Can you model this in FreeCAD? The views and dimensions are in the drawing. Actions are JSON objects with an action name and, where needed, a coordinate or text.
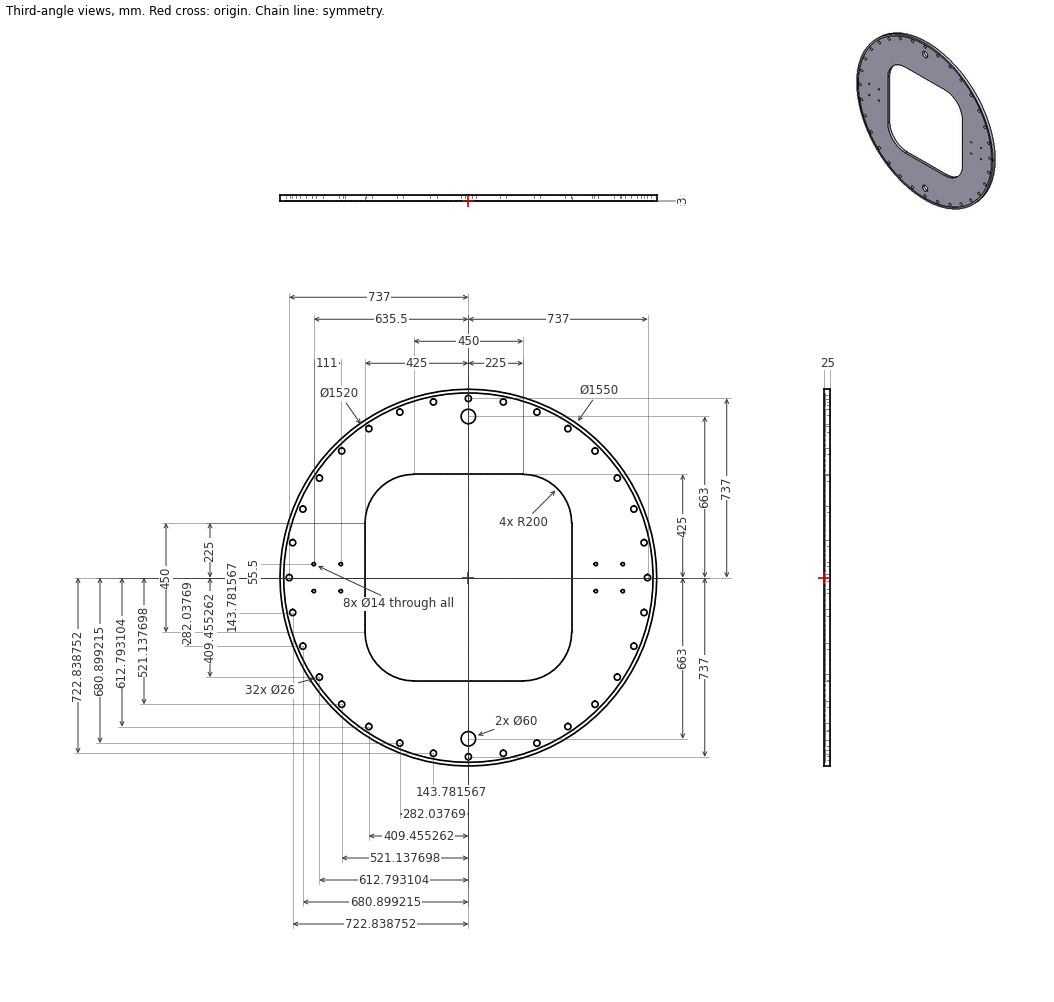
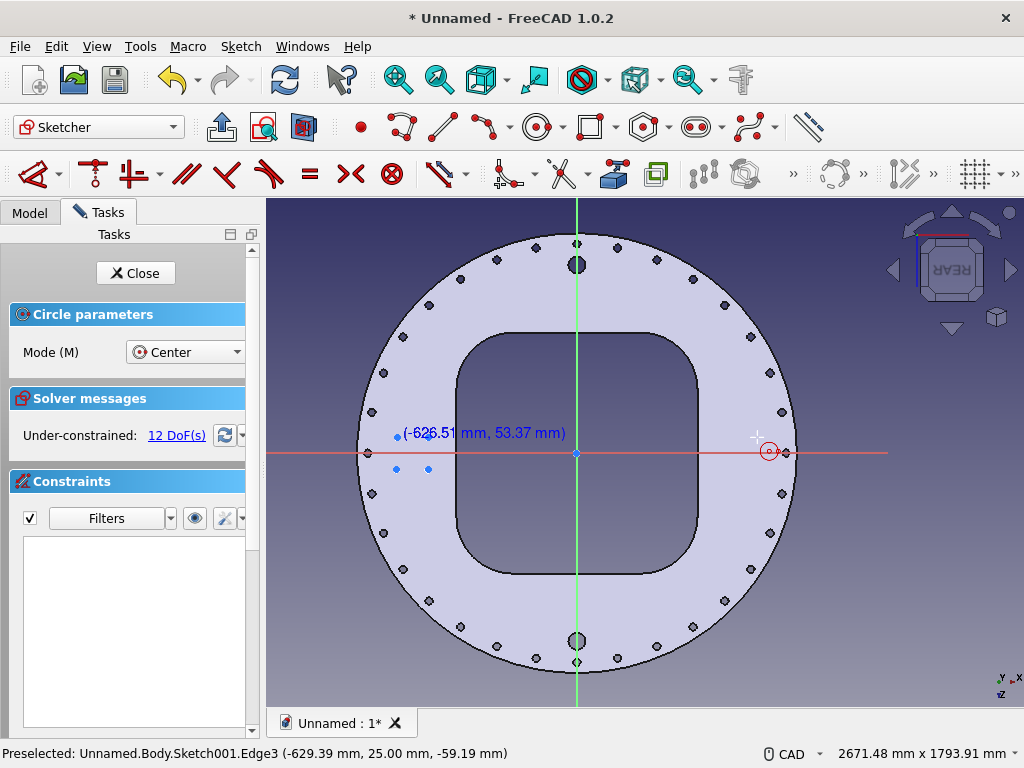
{"action": "left_click", "coordinate": [757, 437]}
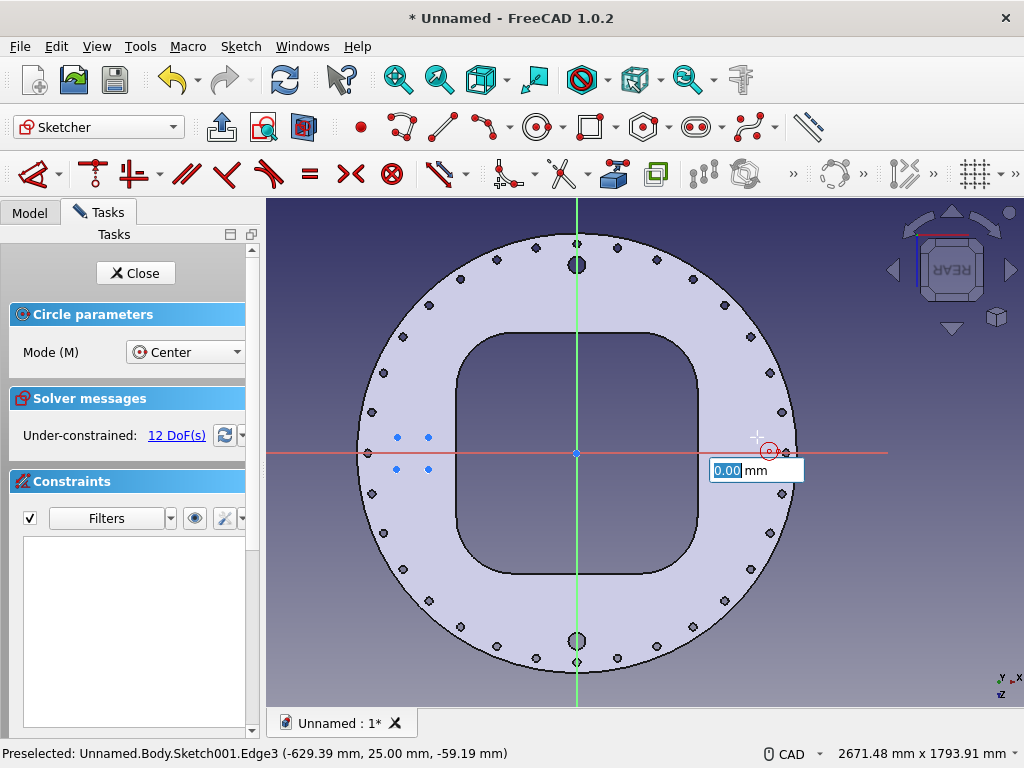
{"action": "scroll", "coordinate": [759, 436], "scroll_direction": "up", "scroll_amount": 11}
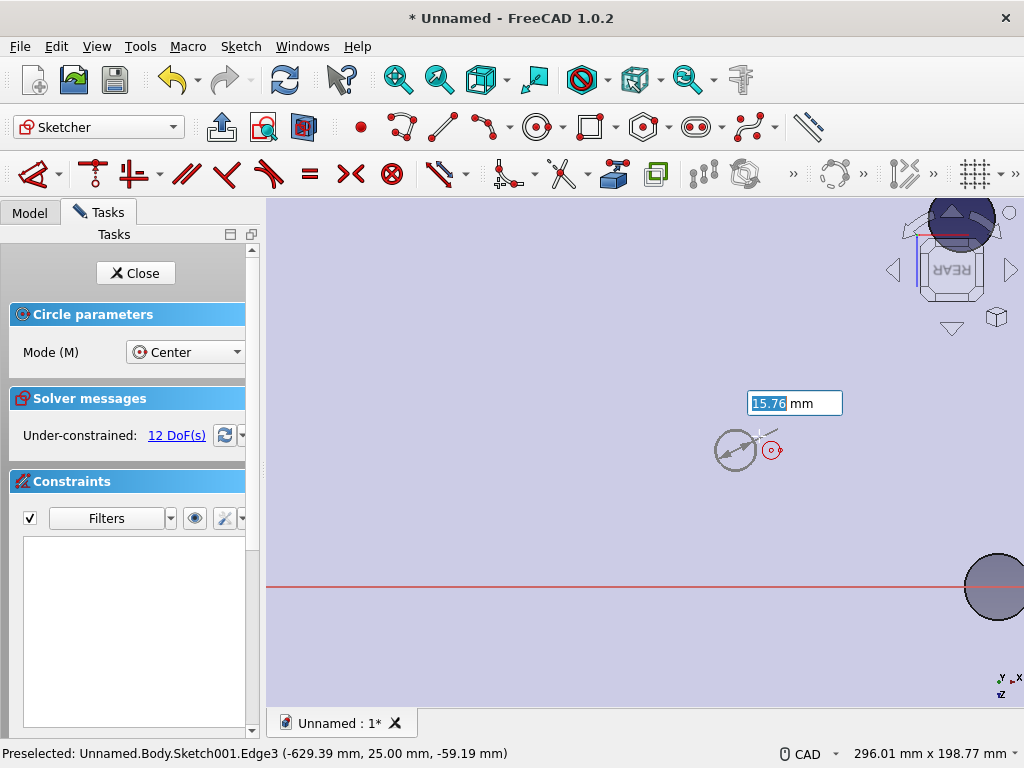
{"action": "left_click", "coordinate": [751, 432]}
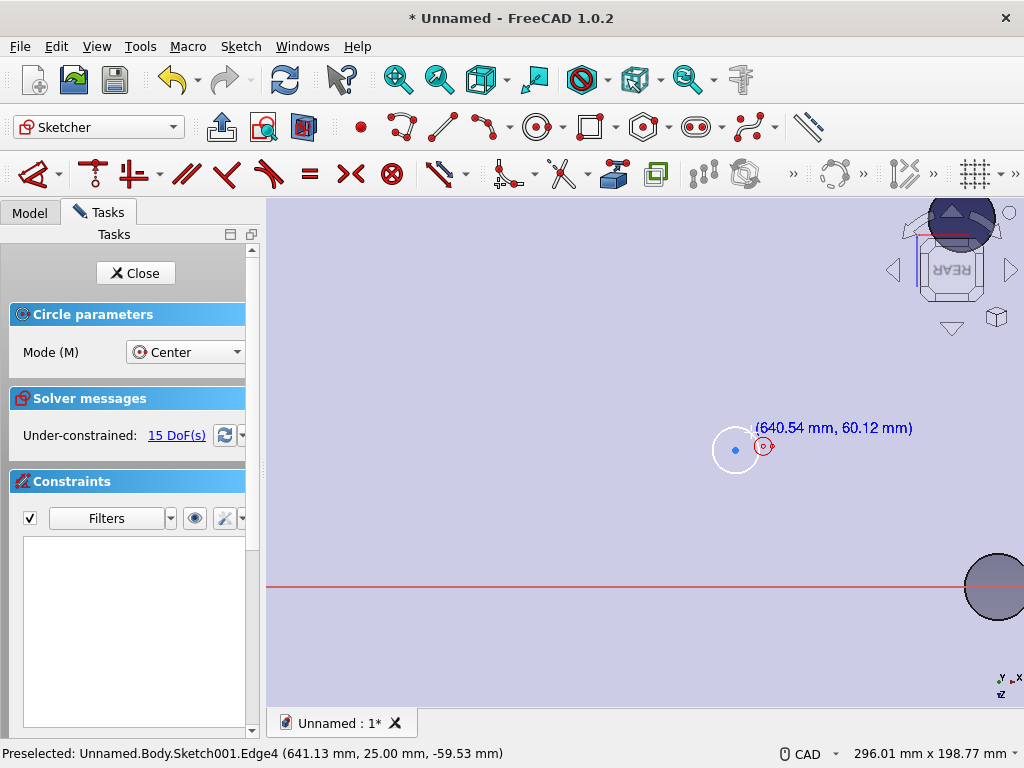
{"action": "scroll", "coordinate": [454, 445], "scroll_direction": "up", "scroll_amount": 2}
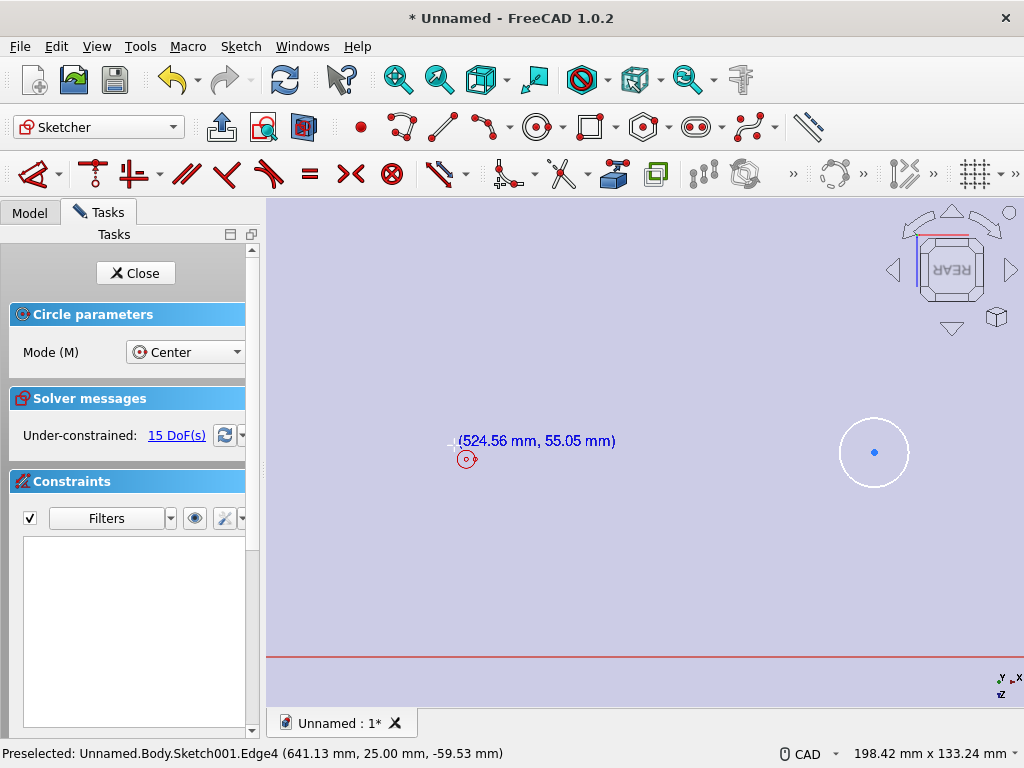
{"action": "scroll", "coordinate": [747, 436], "scroll_direction": "down", "scroll_amount": 13}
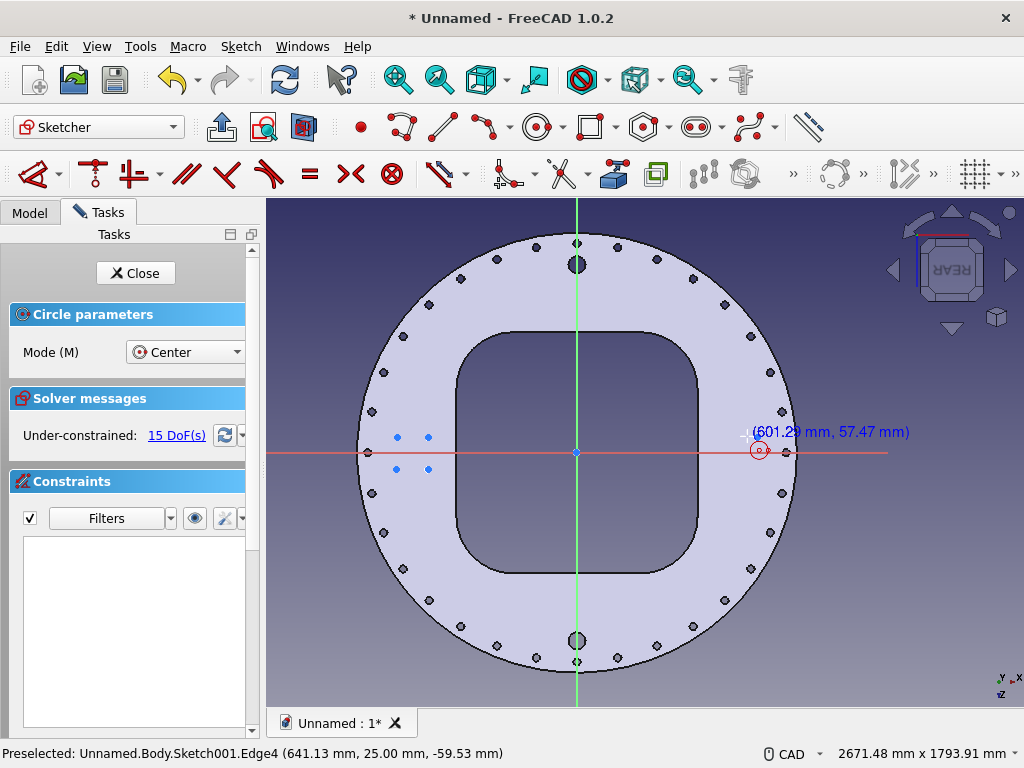
{"action": "left_click", "coordinate": [726, 437]}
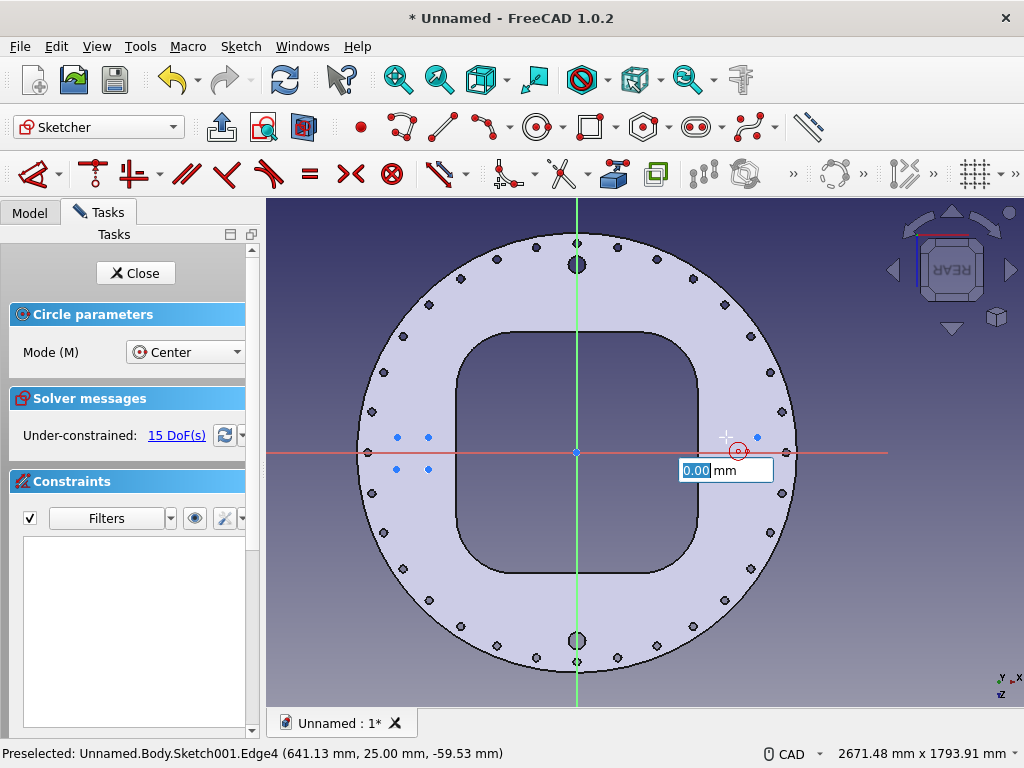
{"action": "scroll", "coordinate": [727, 436], "scroll_direction": "up", "scroll_amount": 11}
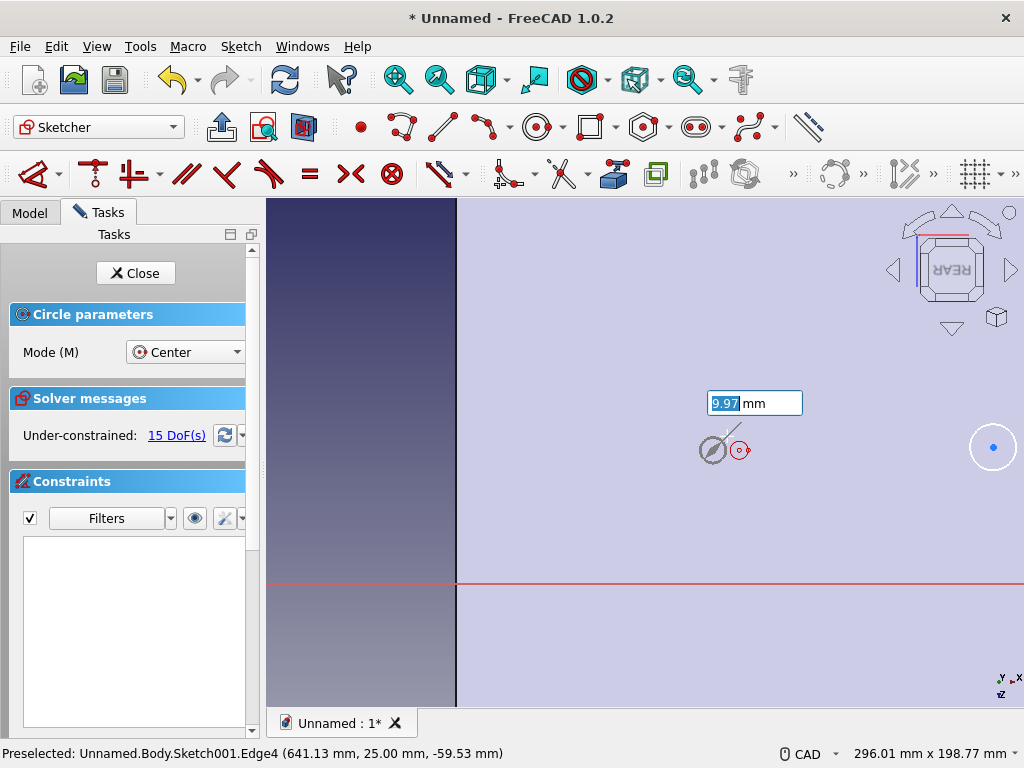
{"action": "left_click", "coordinate": [724, 429]}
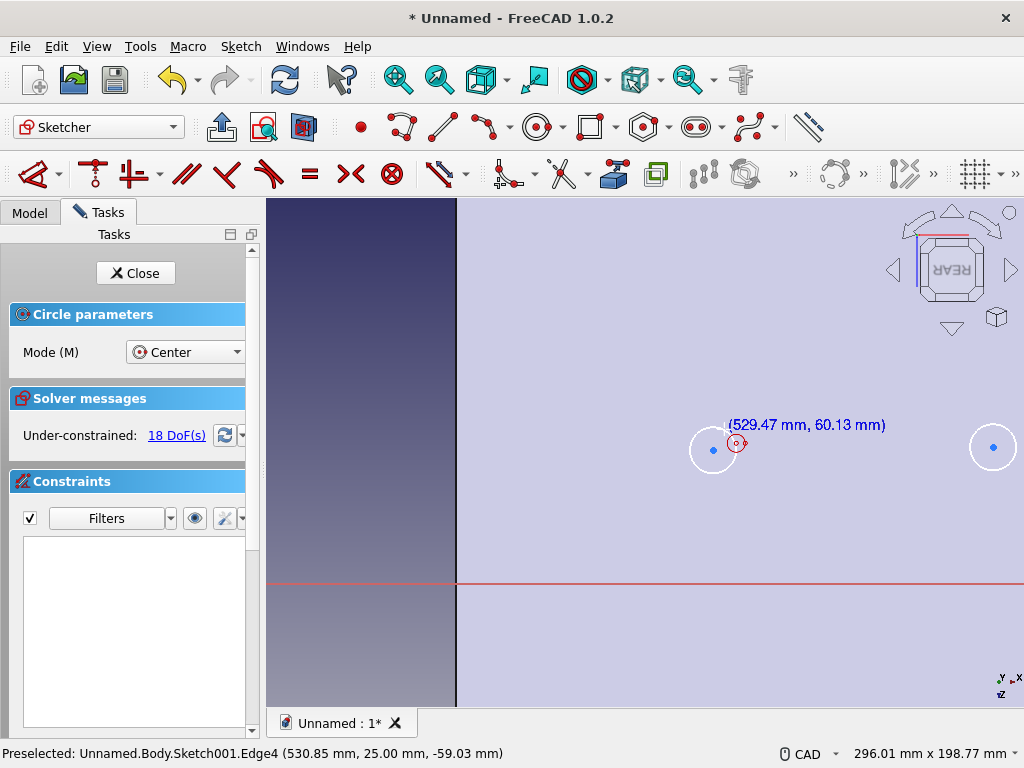
{"action": "scroll", "coordinate": [727, 436], "scroll_direction": "down", "scroll_amount": 11}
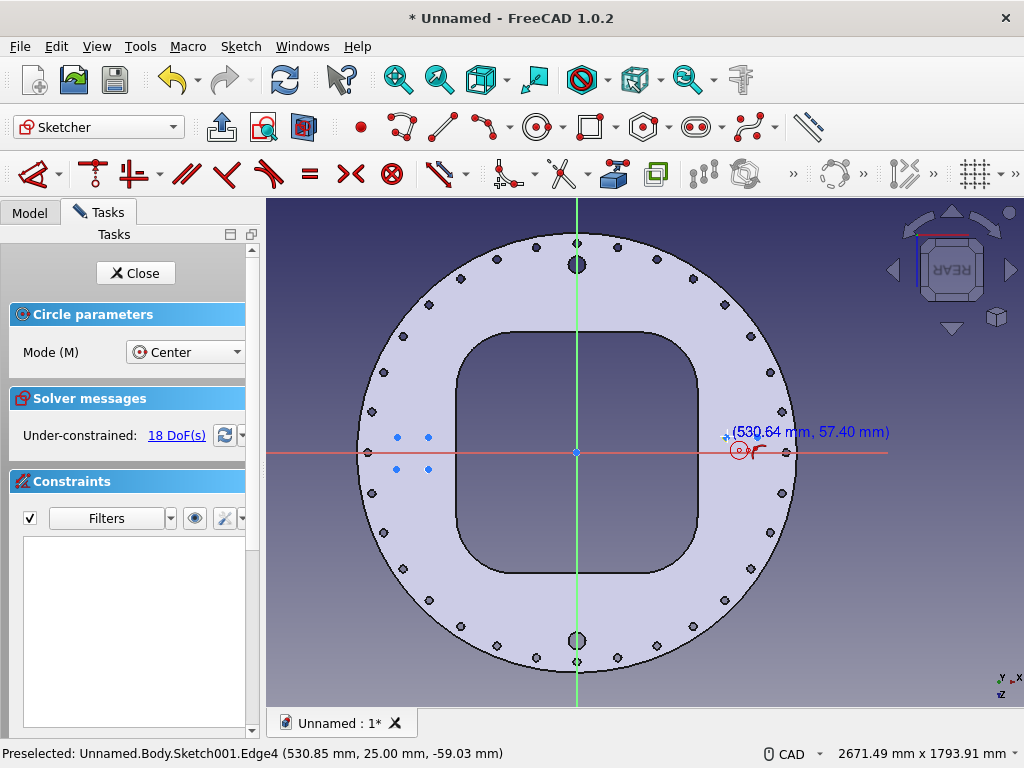
{"action": "scroll", "coordinate": [726, 469], "scroll_direction": "up", "scroll_amount": 13}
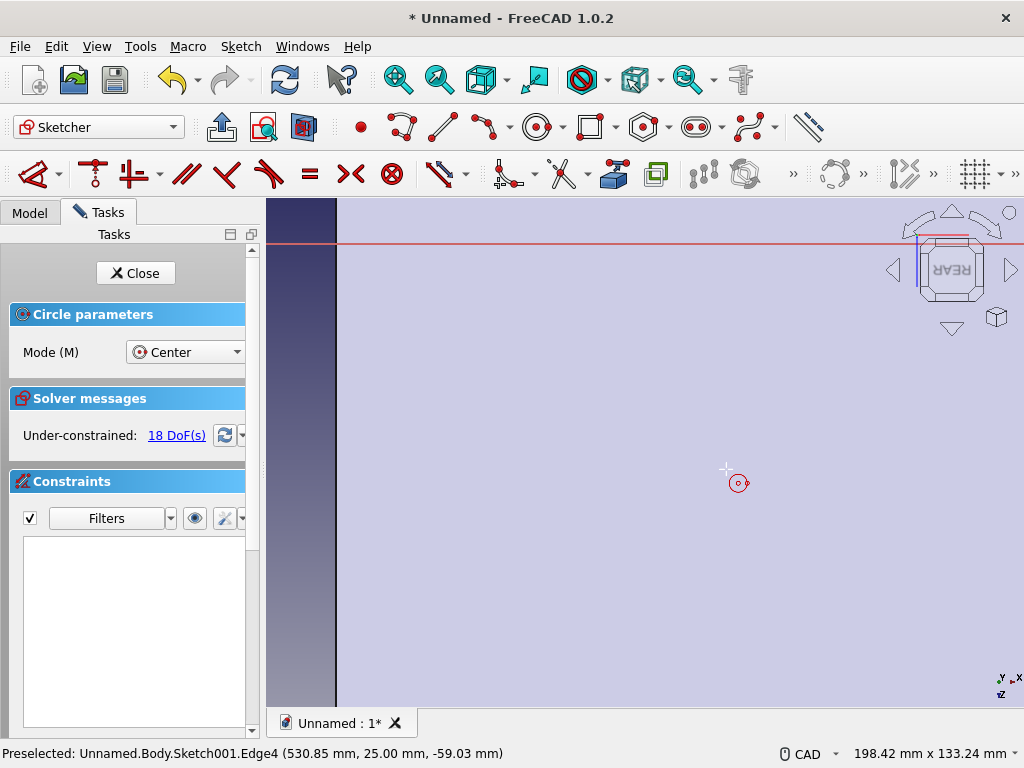
{"action": "scroll", "coordinate": [726, 469], "scroll_direction": "down", "scroll_amount": 13}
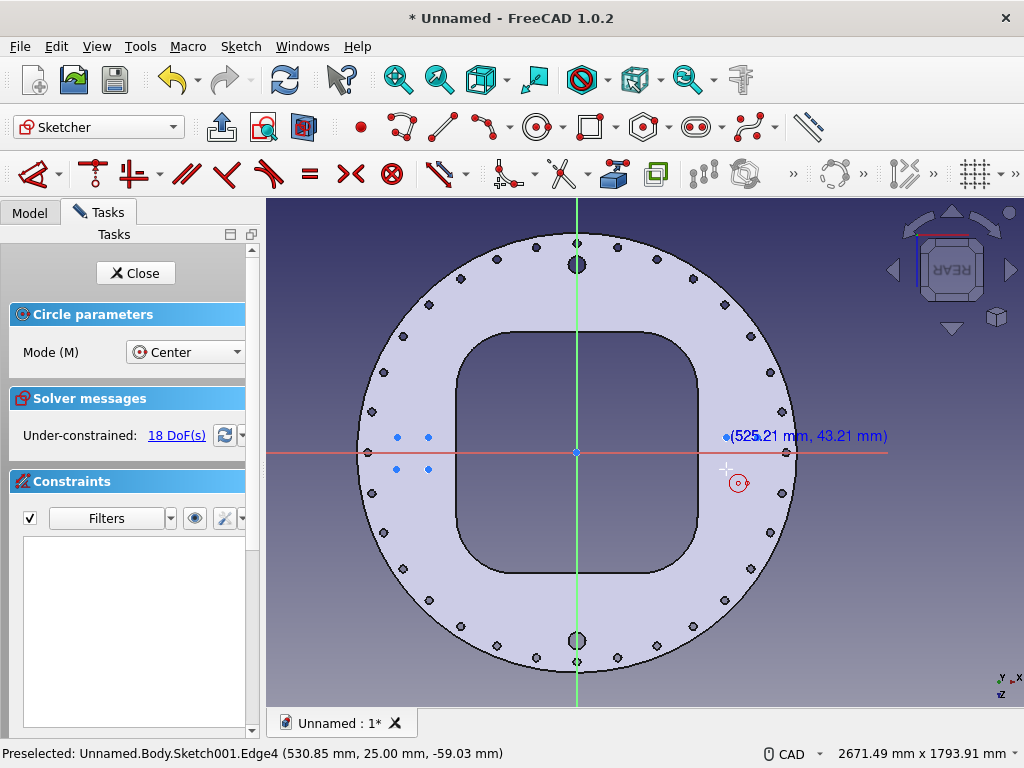
{"action": "left_click", "coordinate": [726, 469]}